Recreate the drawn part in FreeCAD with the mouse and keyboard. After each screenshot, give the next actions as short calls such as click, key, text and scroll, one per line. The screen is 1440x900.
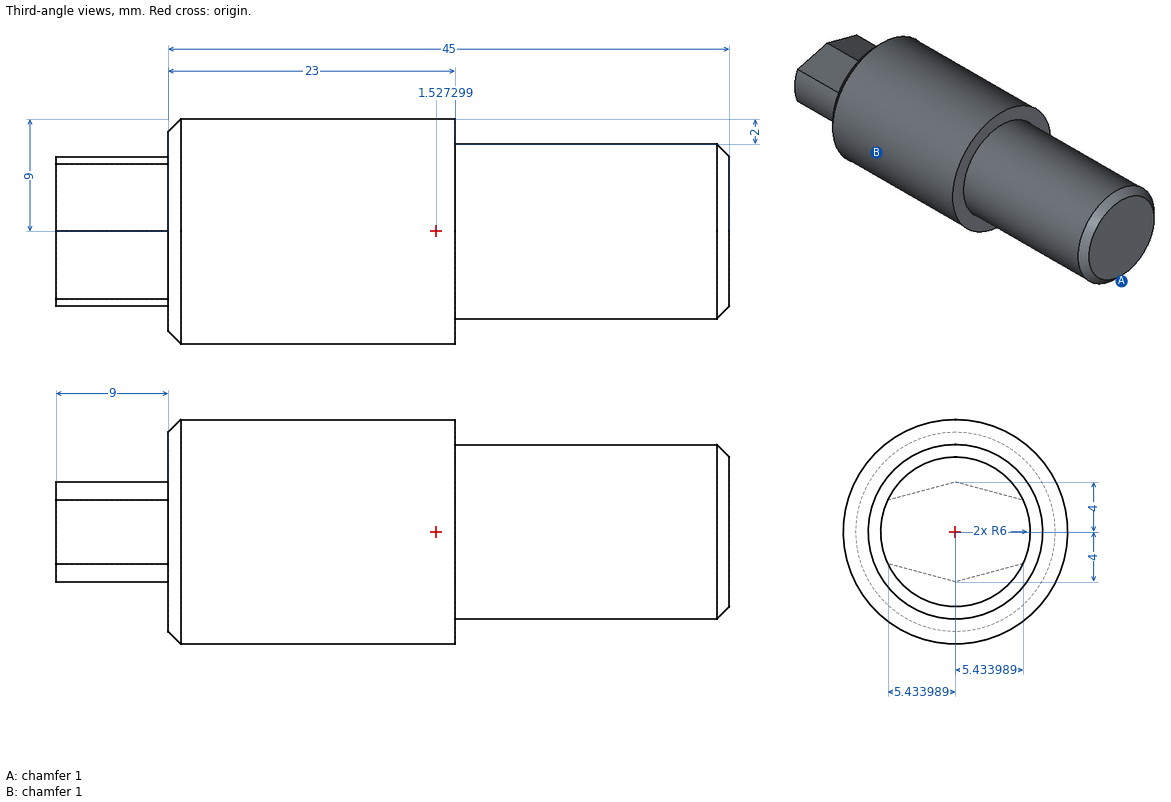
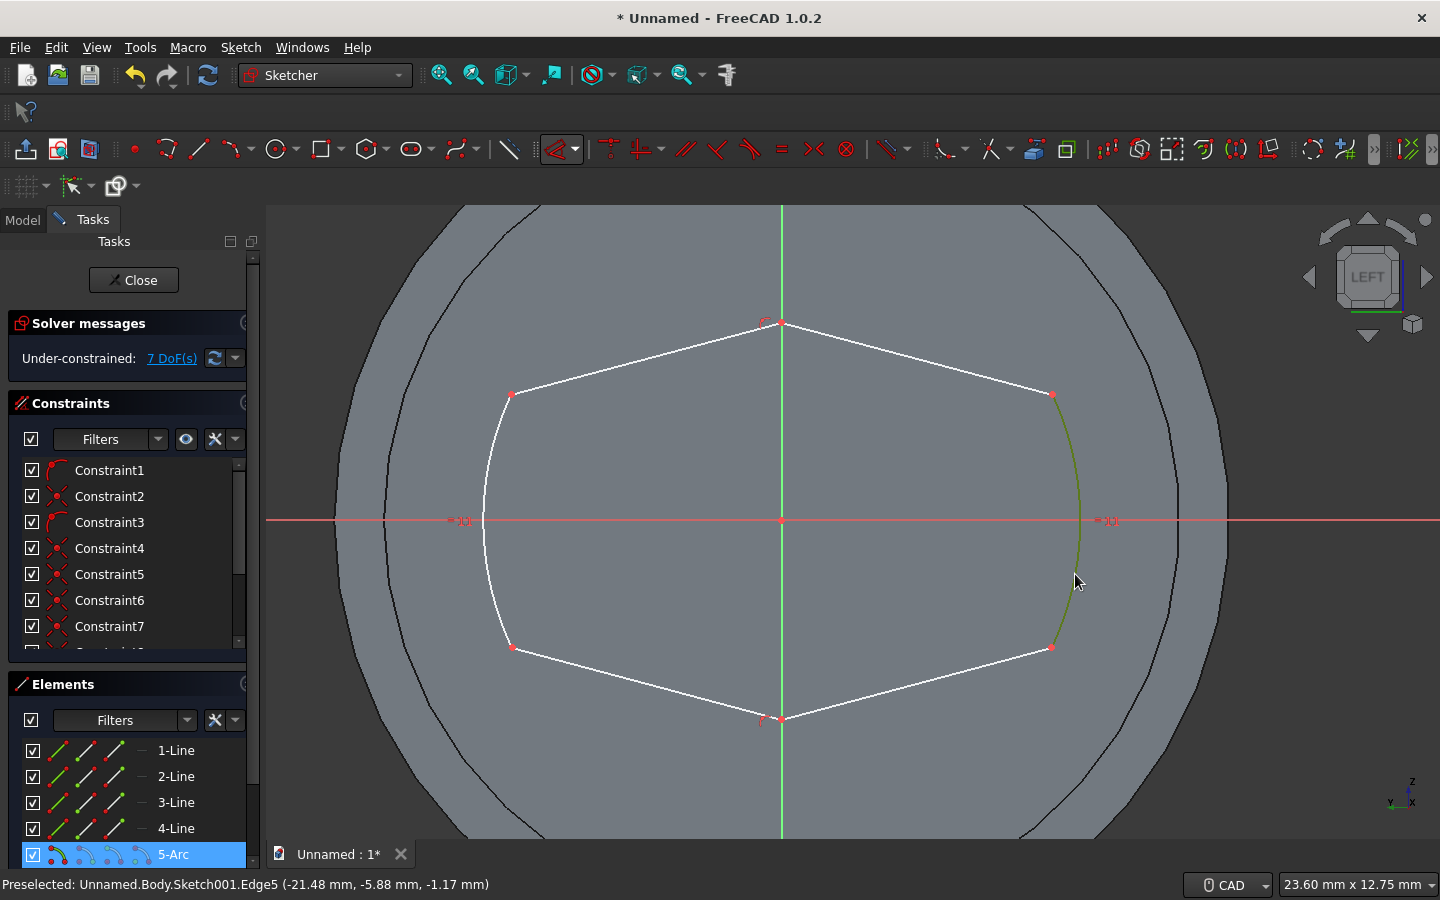
key(k)
key(r)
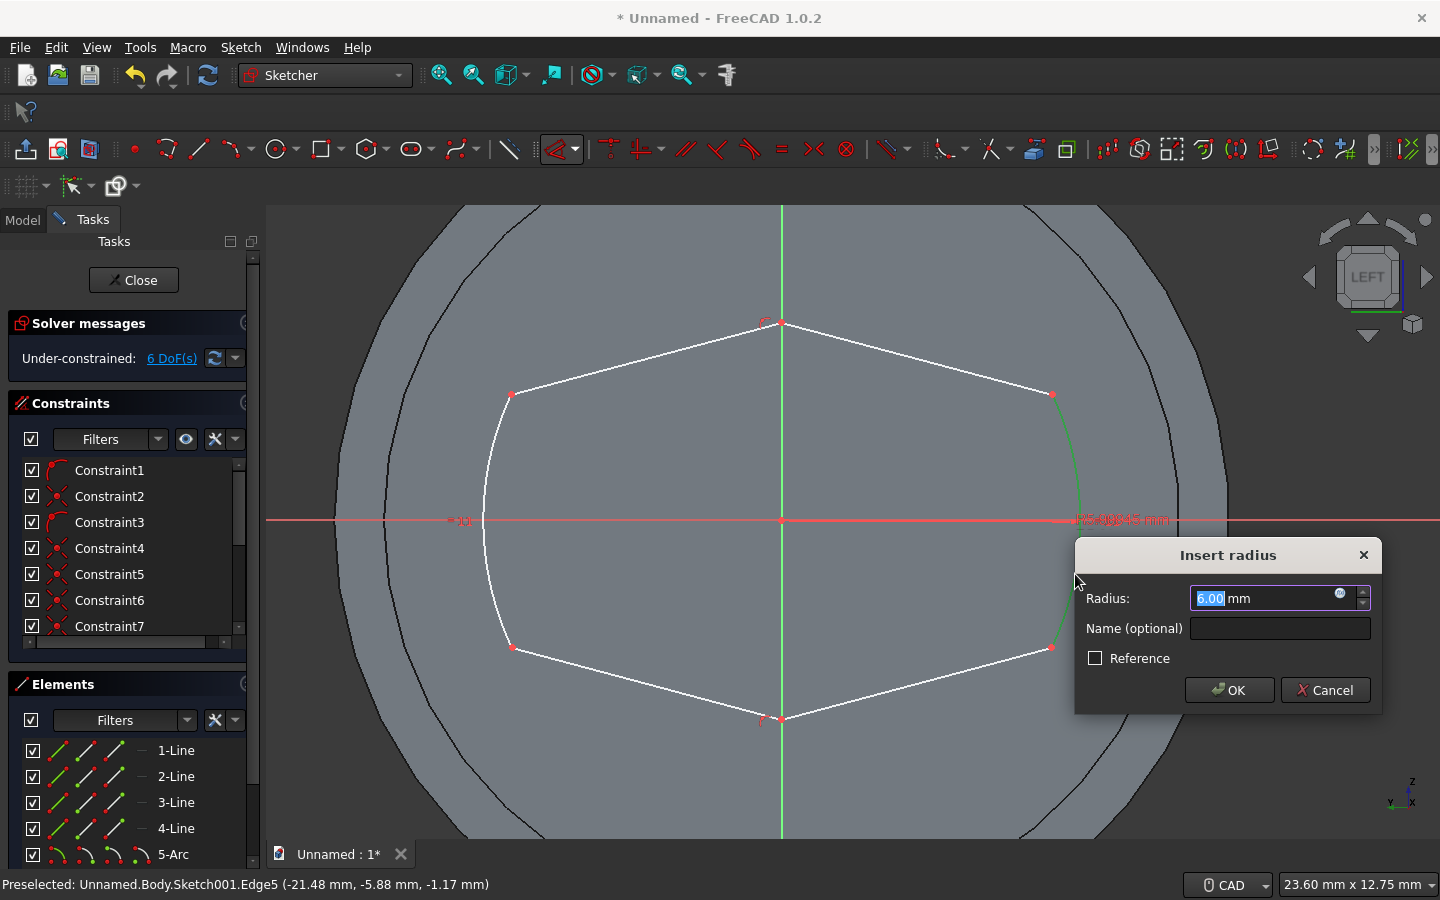
text(6)
key(Return)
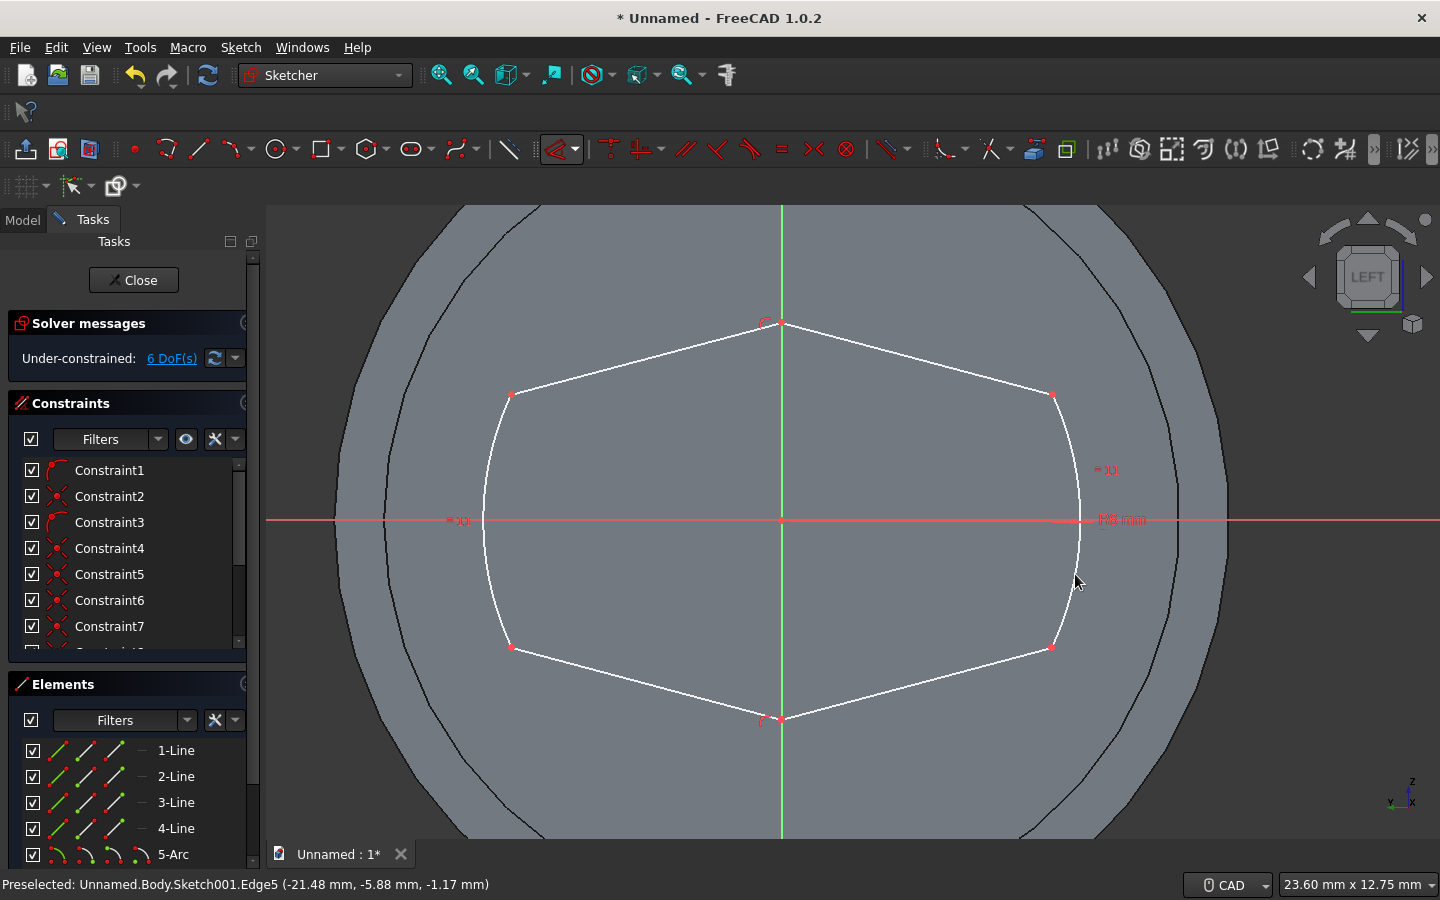
click(782, 720)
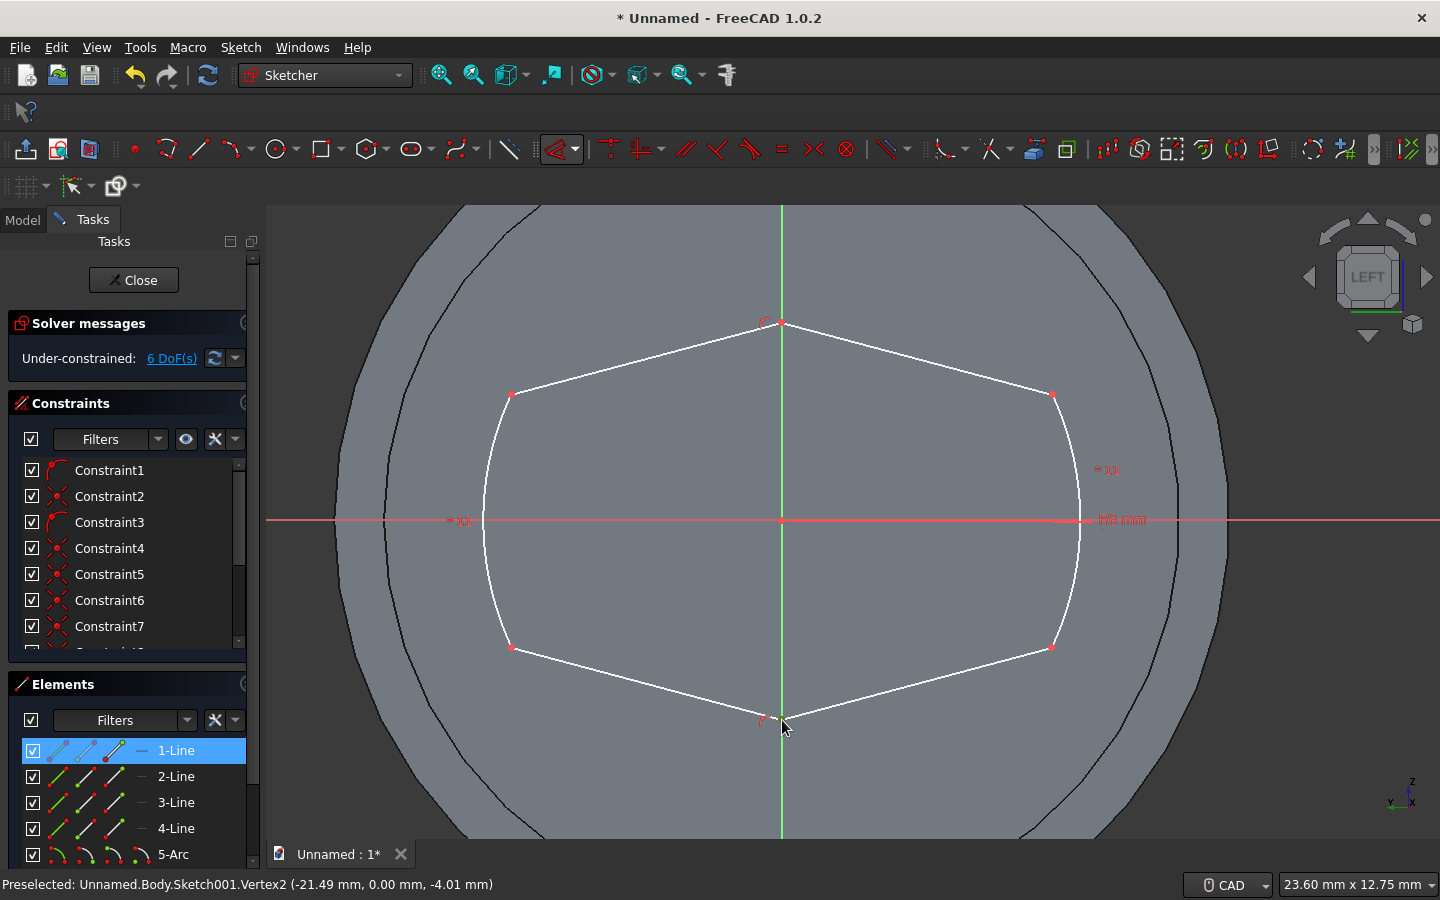
click(578, 150)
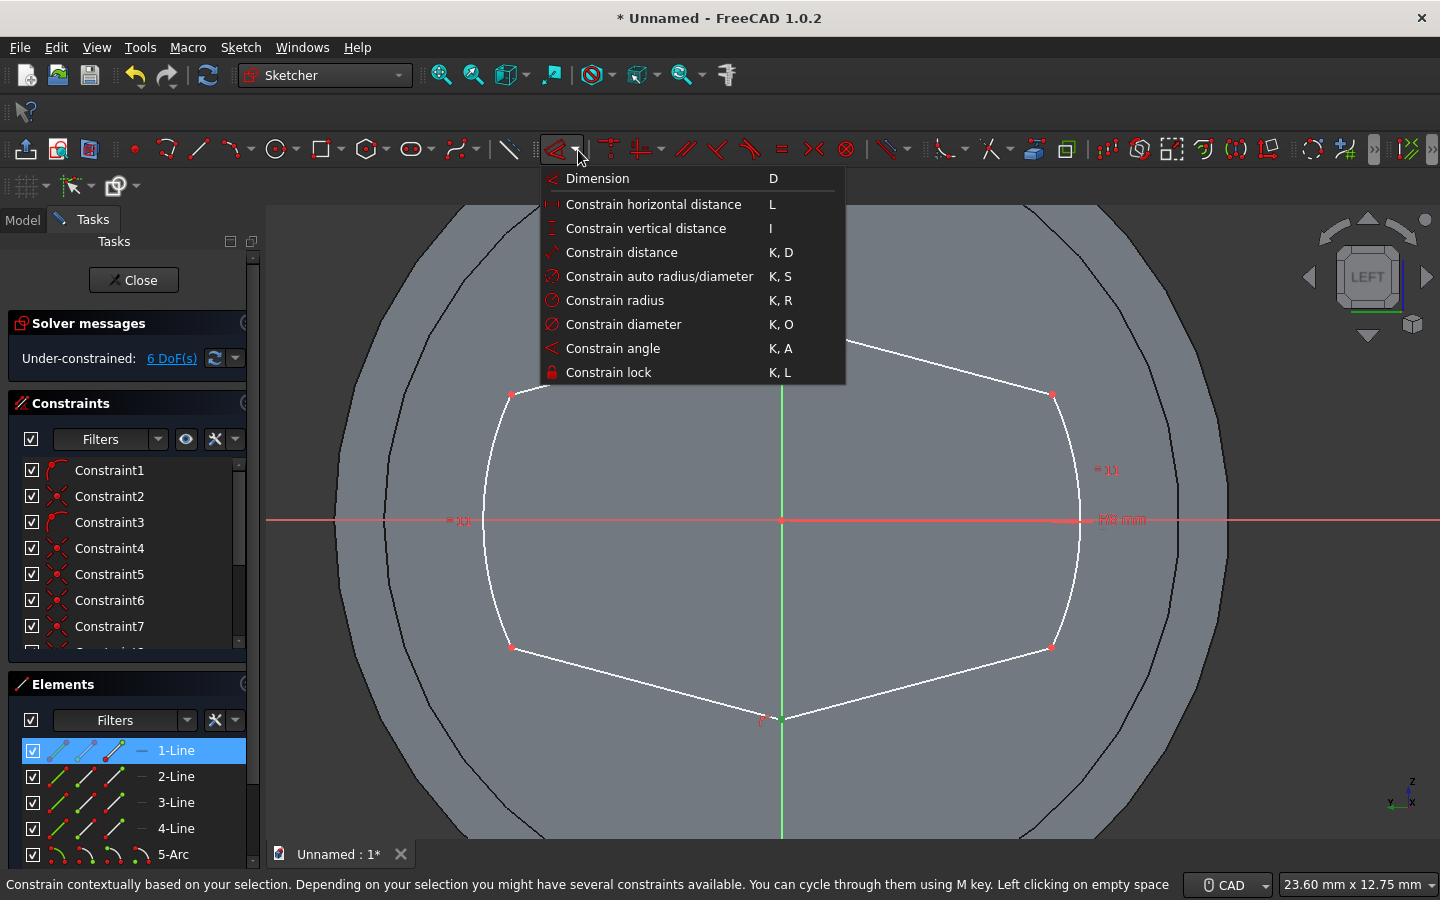
click(693, 228)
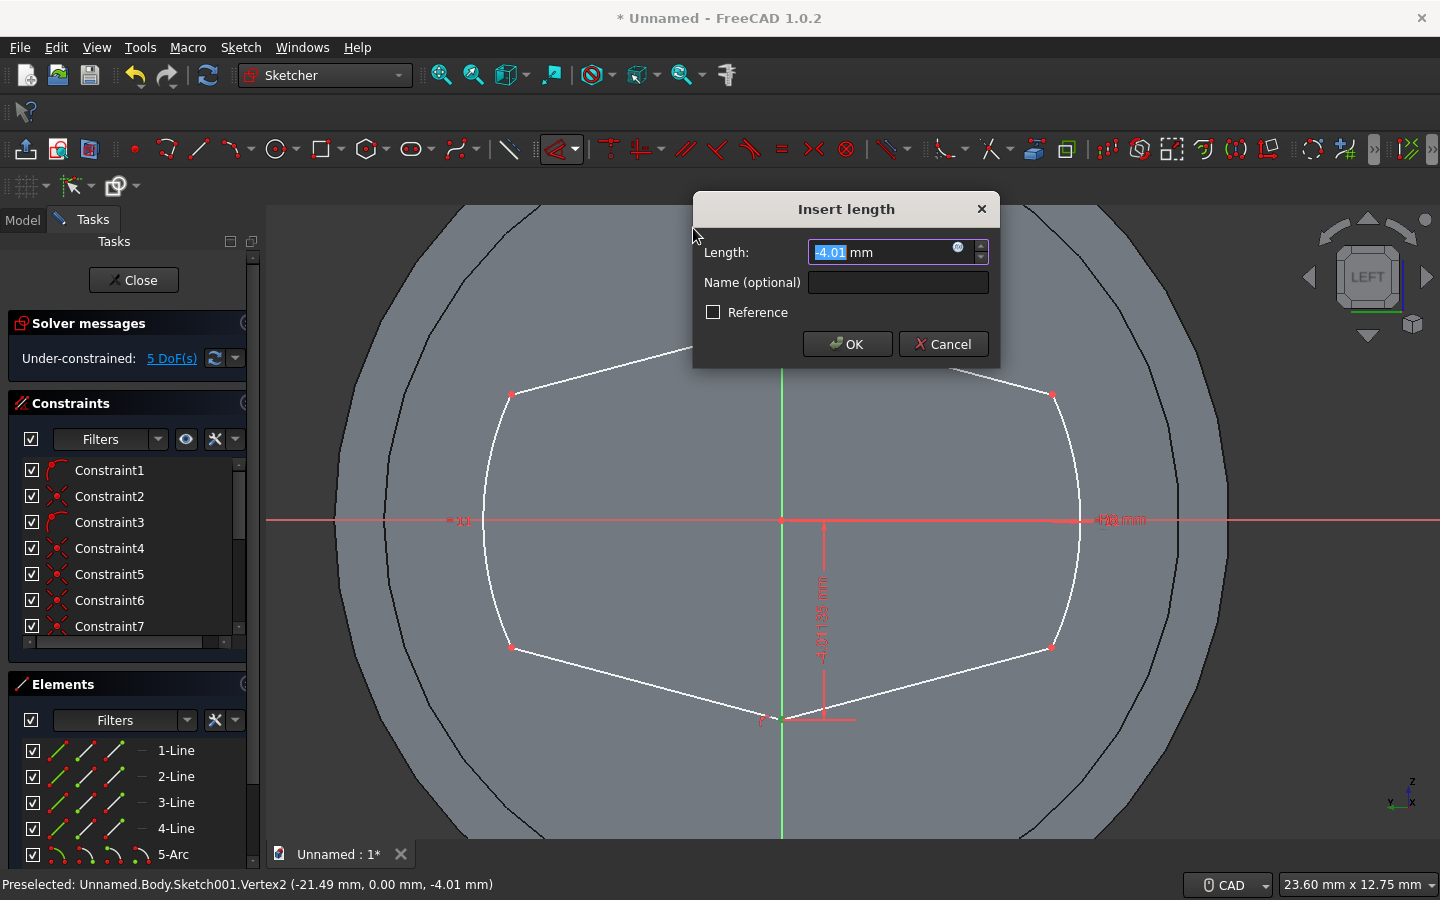
text(-4)
key(Return)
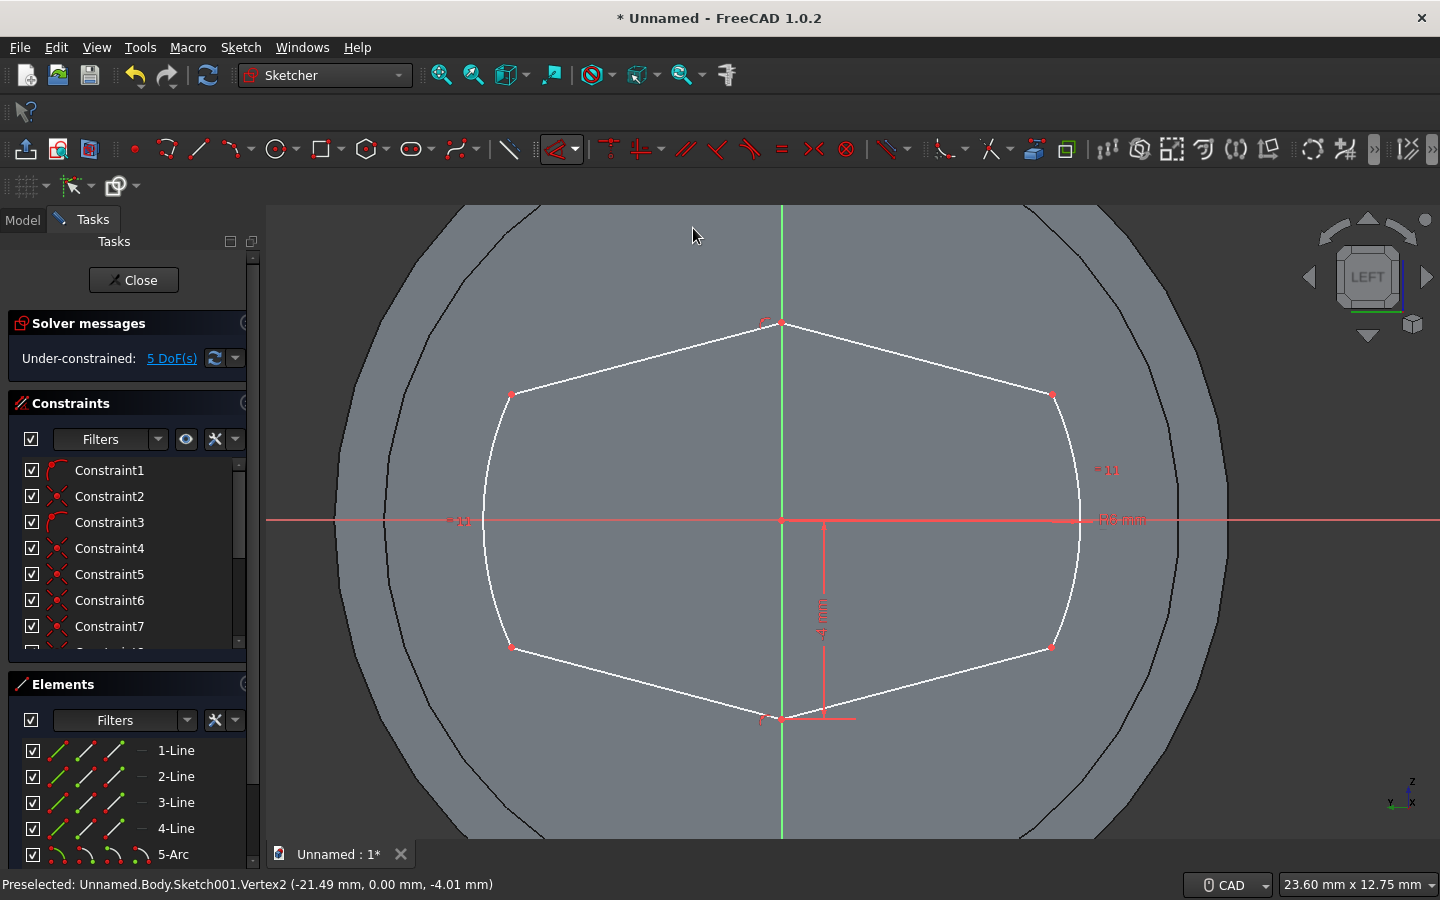
click(782, 323)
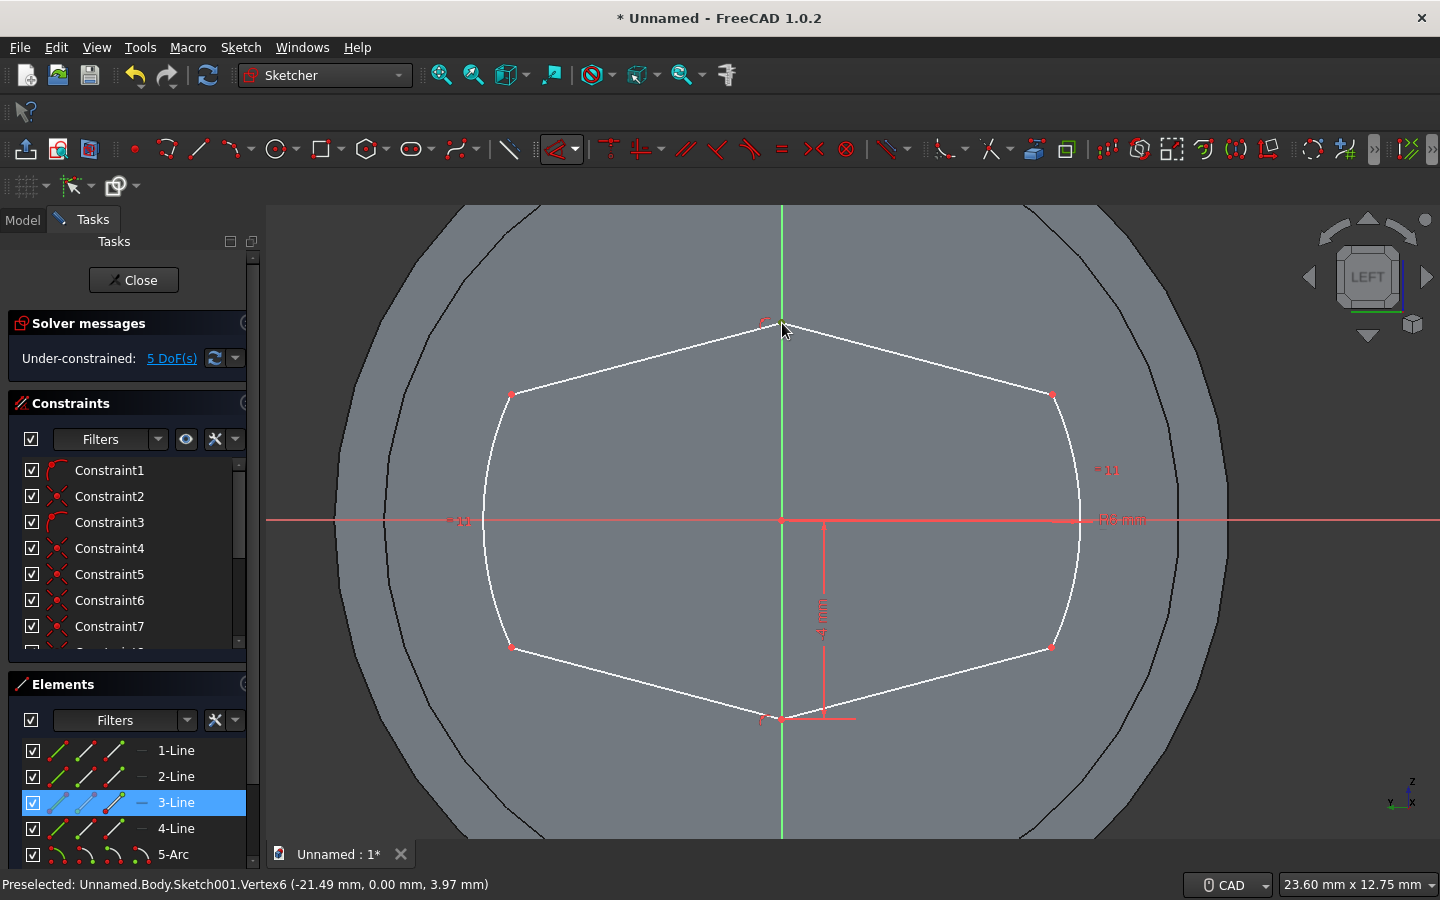
click(578, 150)